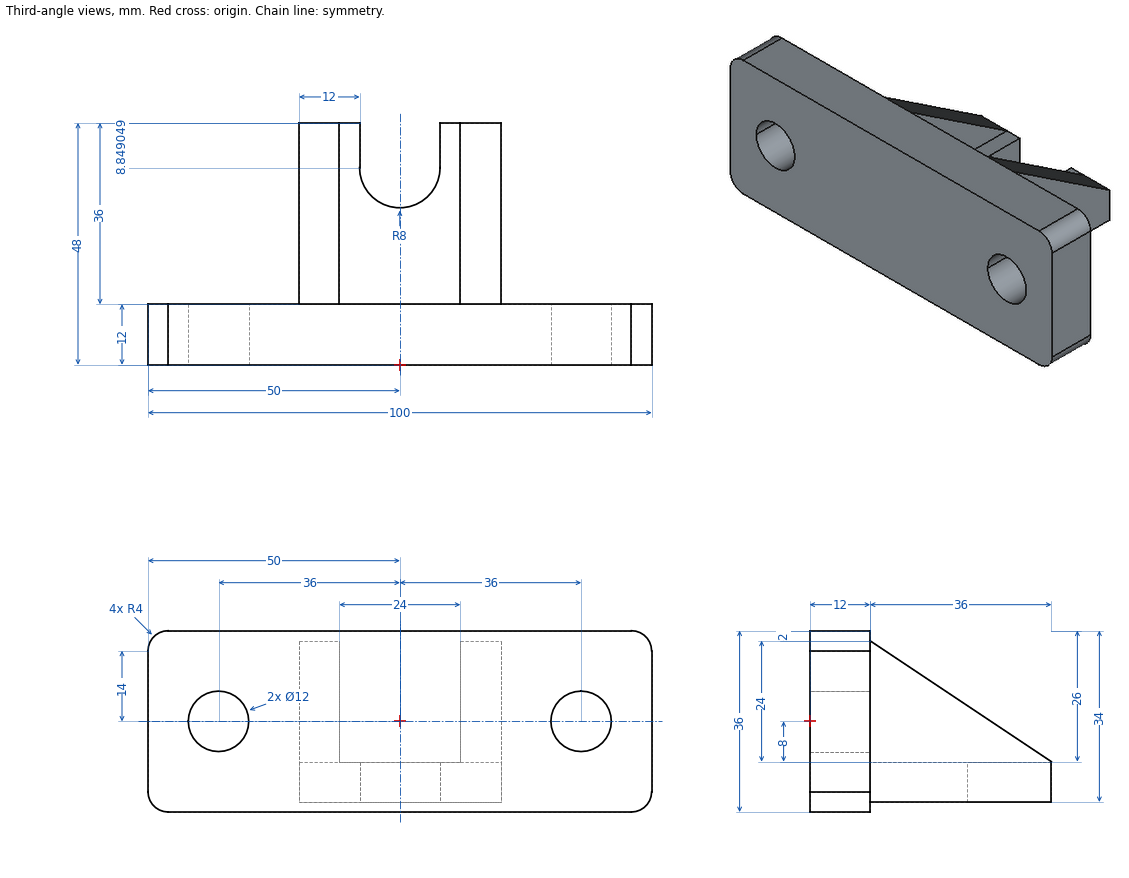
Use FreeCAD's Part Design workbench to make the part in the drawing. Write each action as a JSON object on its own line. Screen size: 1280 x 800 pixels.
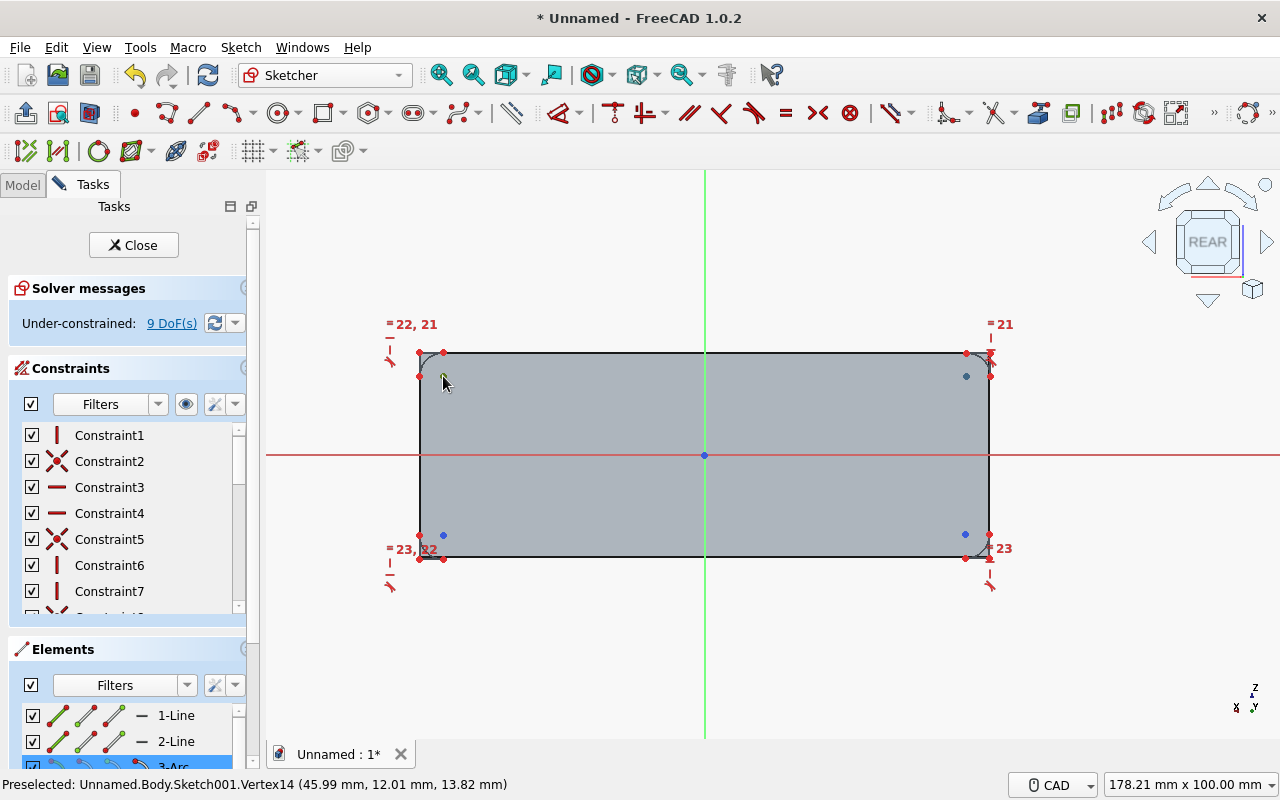
{"action": "left_click", "coordinate": [705, 674]}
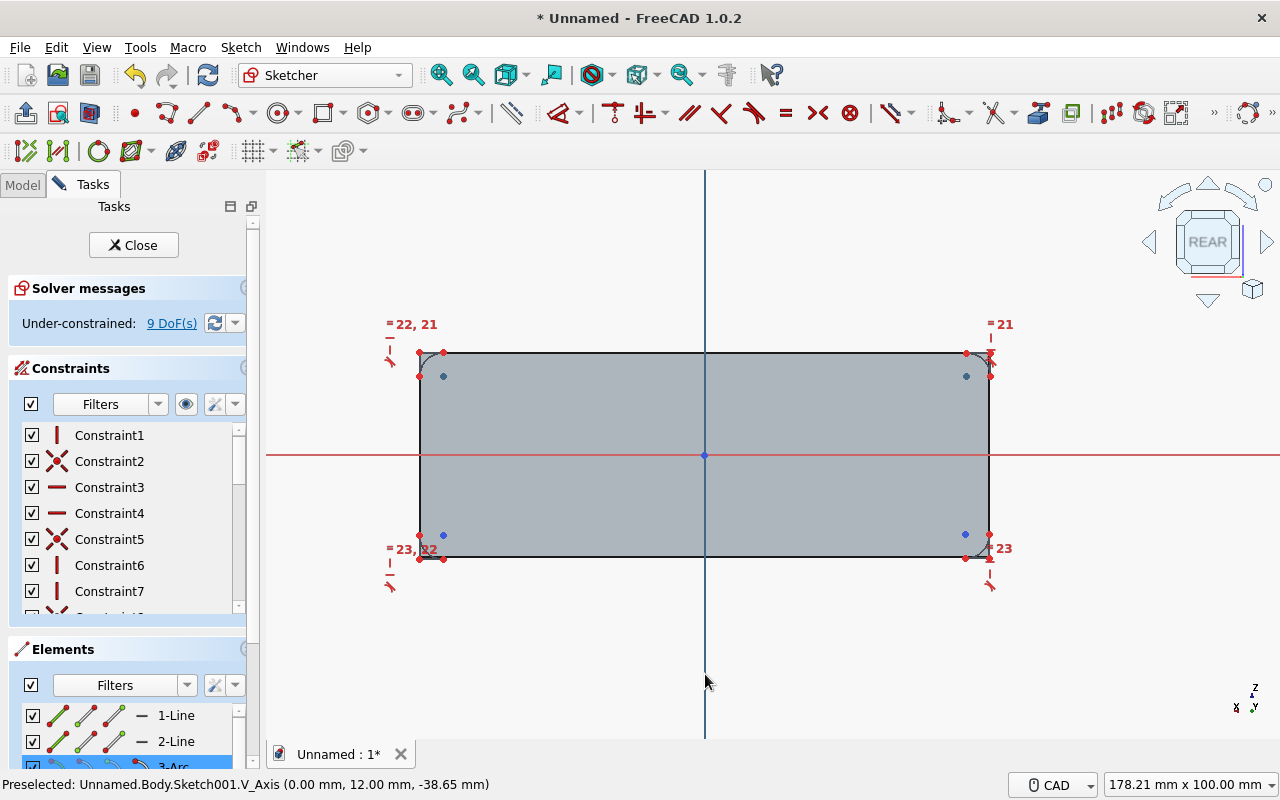
{"action": "left_click", "coordinate": [818, 114]}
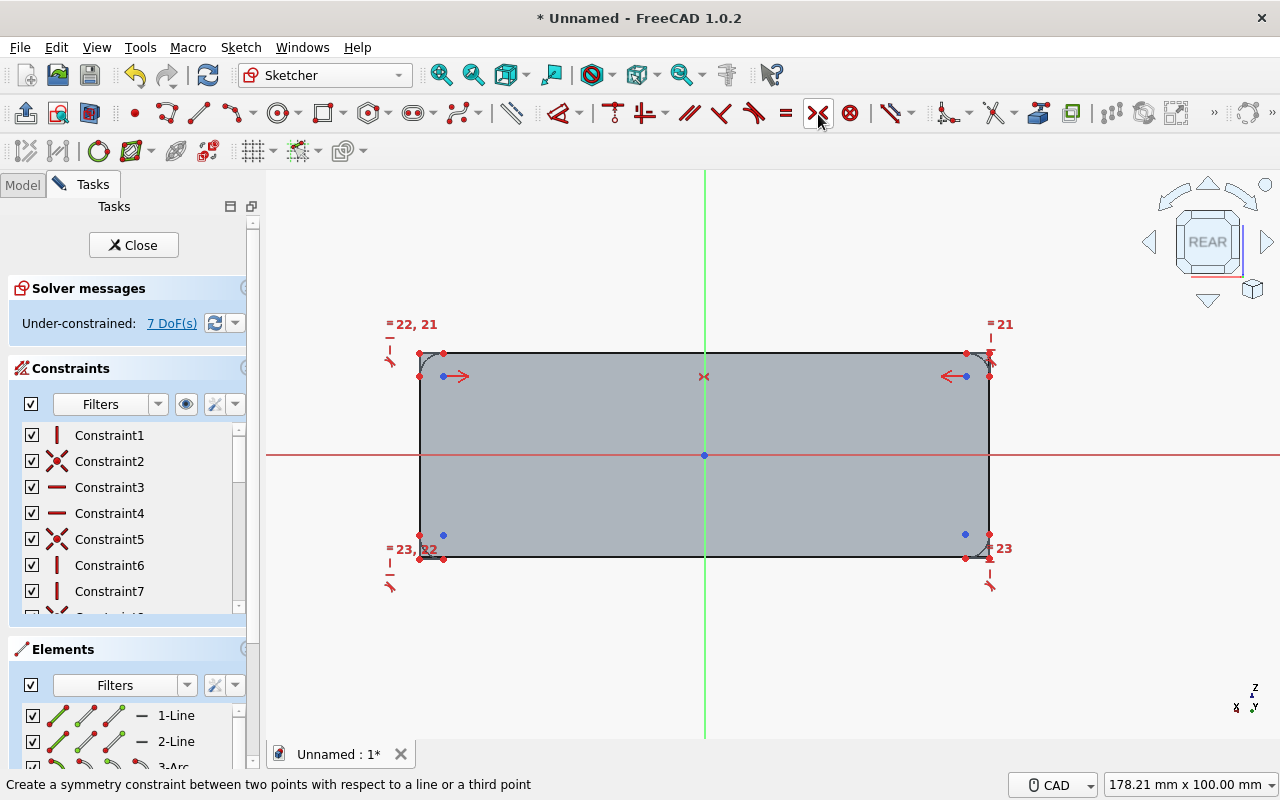
{"action": "left_click", "coordinate": [443, 376]}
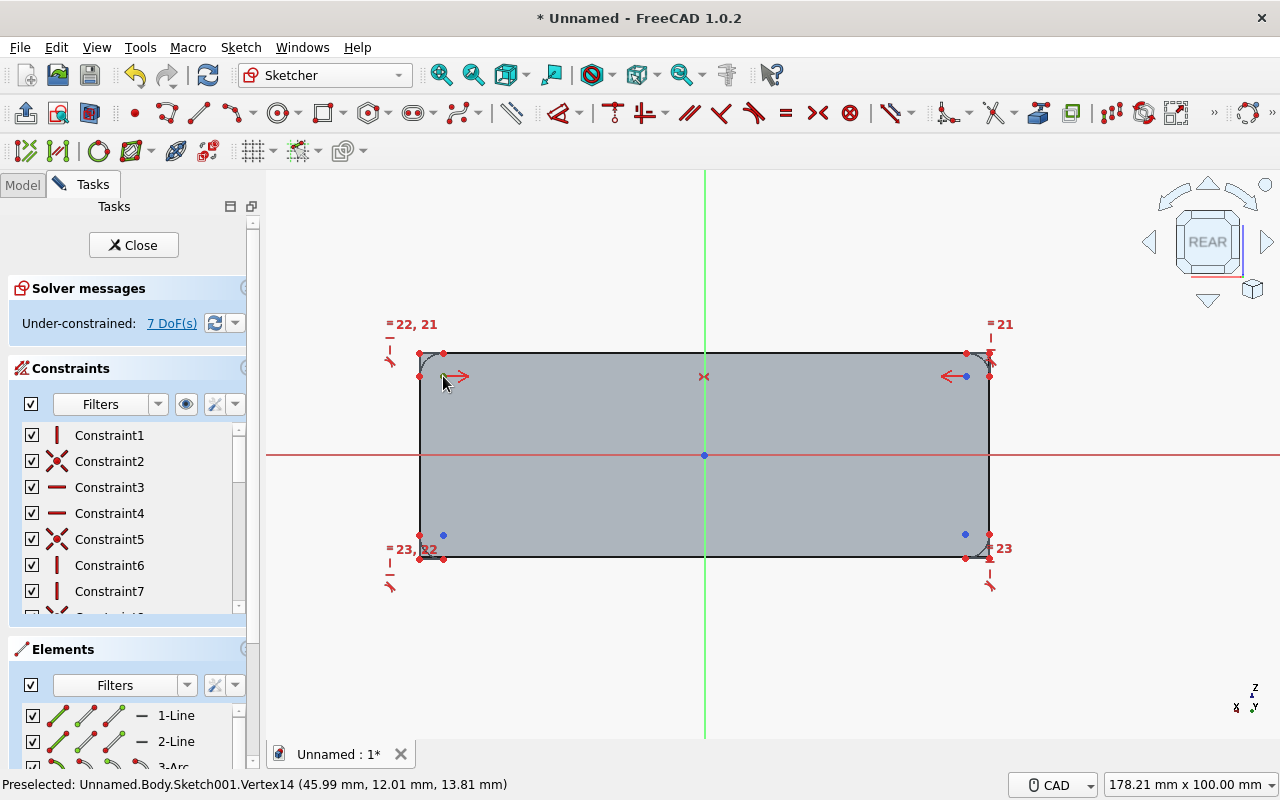
{"action": "left_click", "coordinate": [443, 536]}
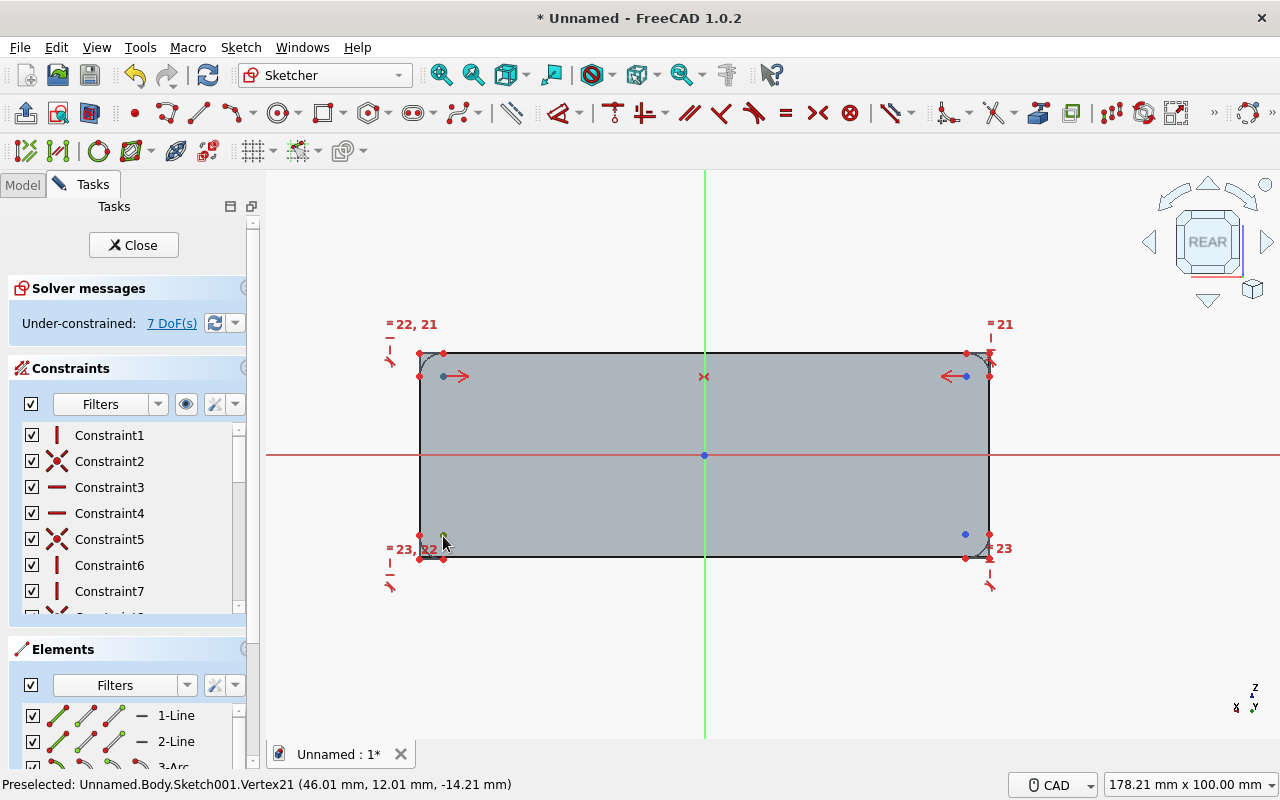
{"action": "left_click", "coordinate": [353, 455]}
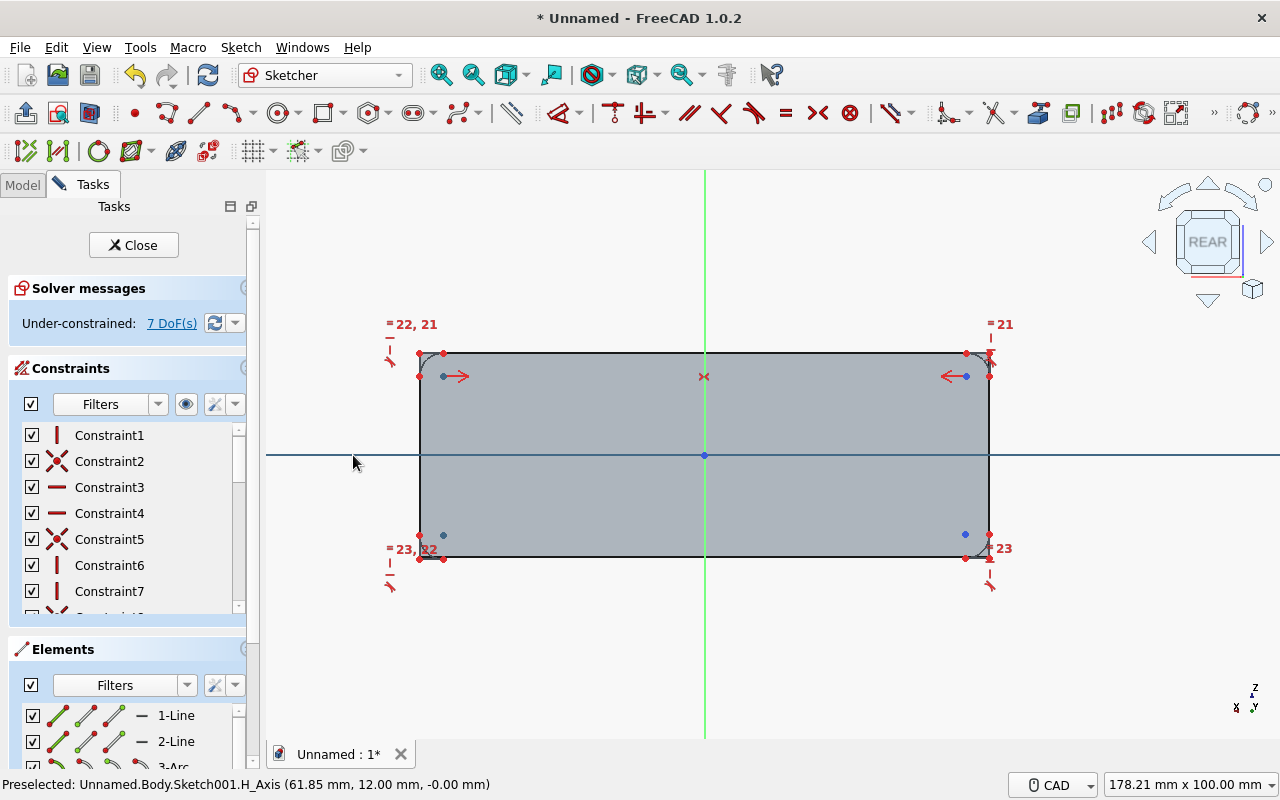
{"action": "left_click", "coordinate": [818, 114]}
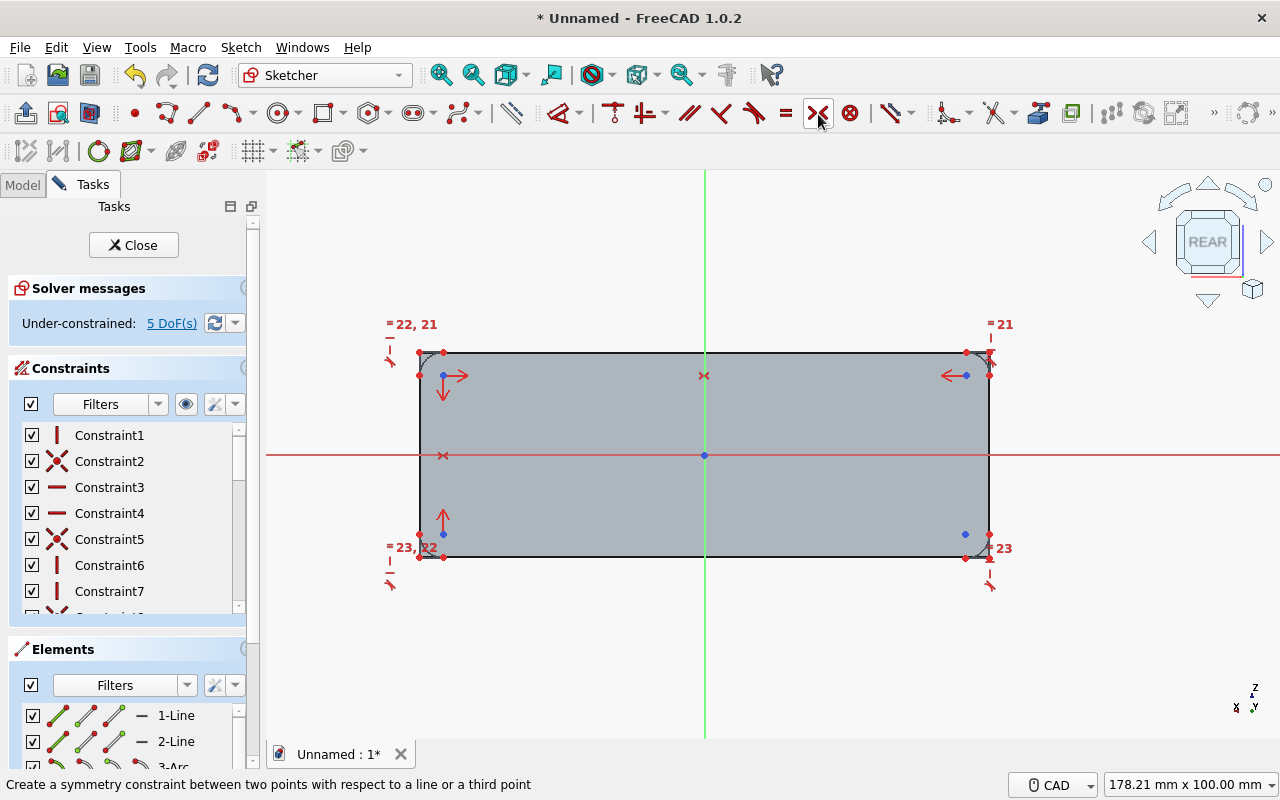
{"action": "left_click", "coordinate": [967, 376]}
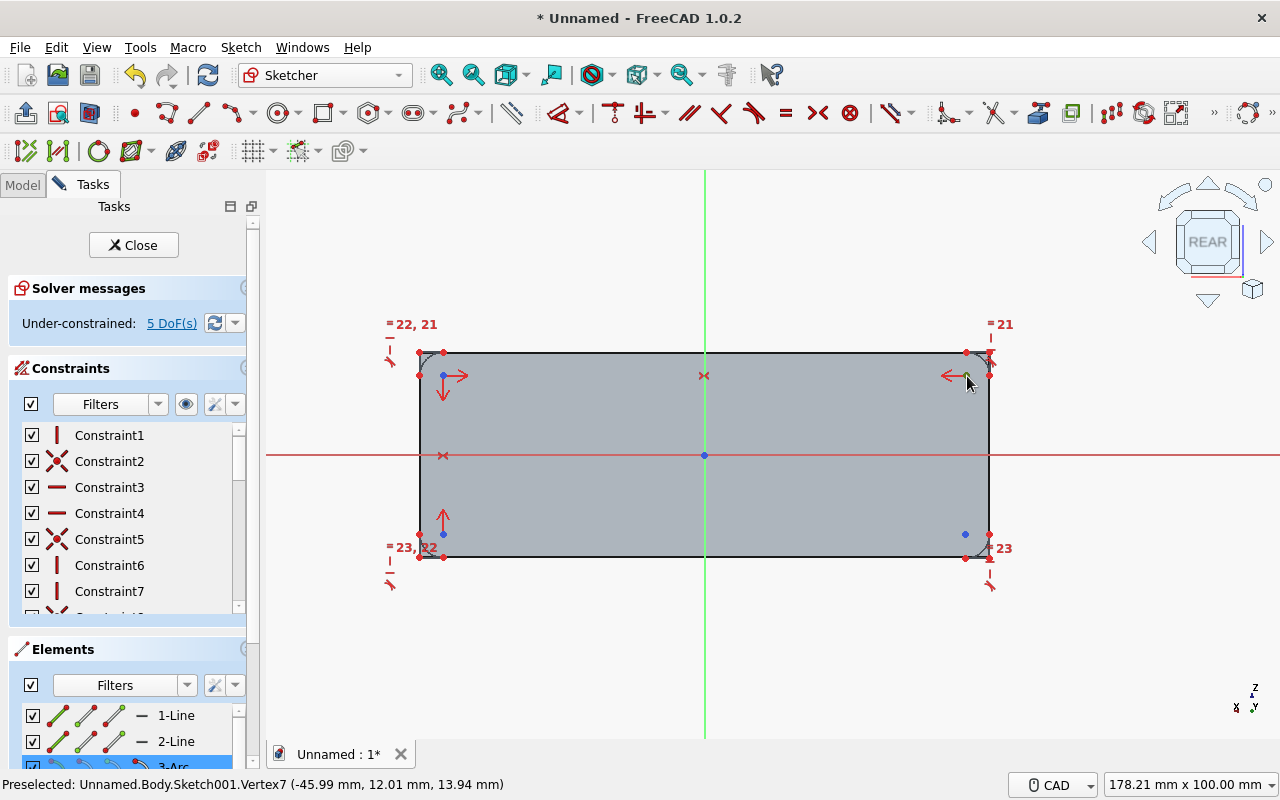
{"action": "left_click", "coordinate": [966, 535]}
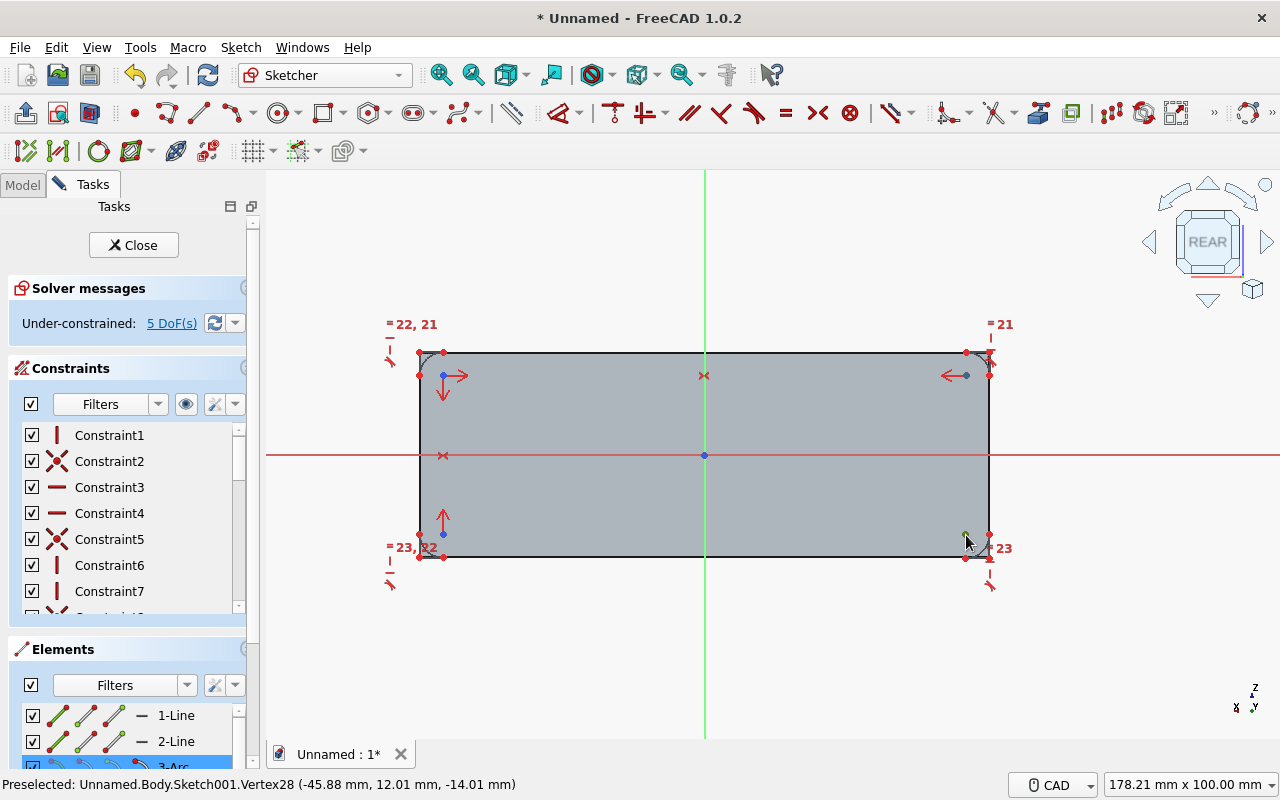
{"action": "left_click", "coordinate": [353, 455]}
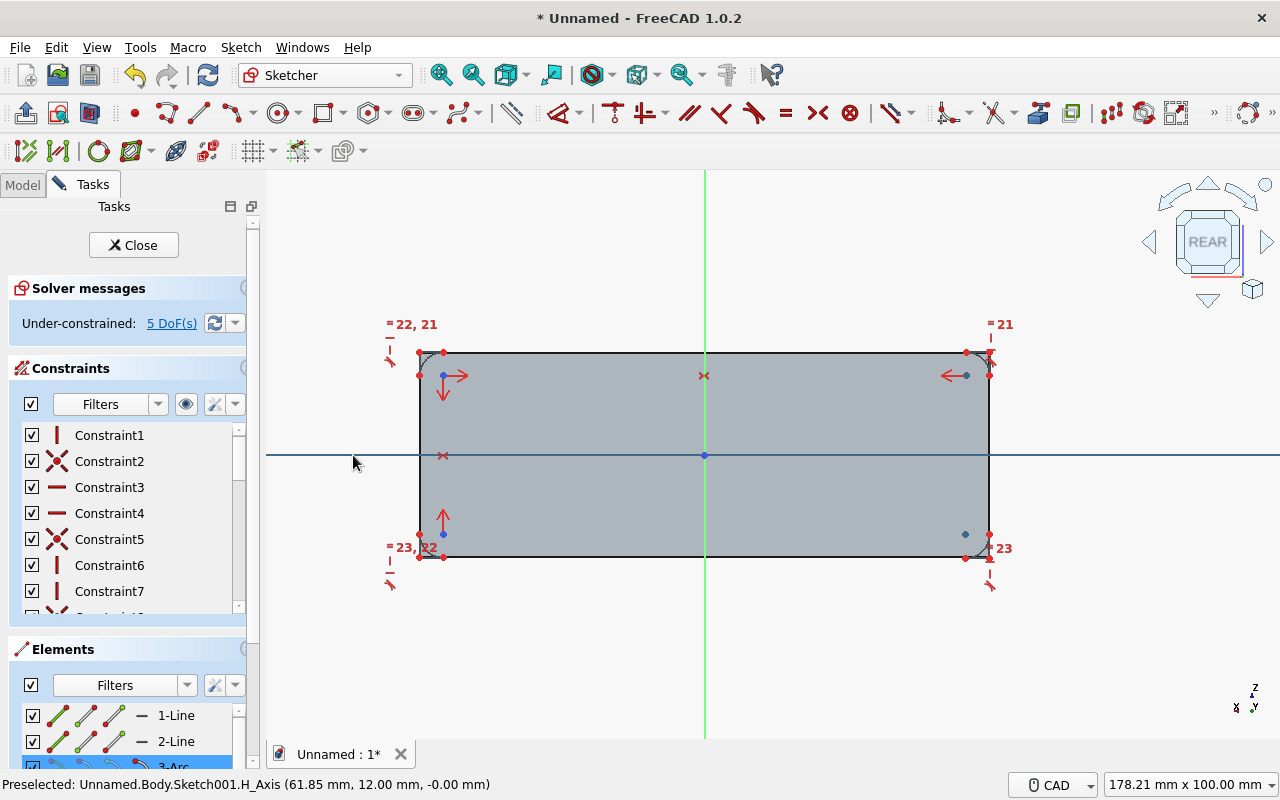
{"action": "left_click", "coordinate": [818, 114]}